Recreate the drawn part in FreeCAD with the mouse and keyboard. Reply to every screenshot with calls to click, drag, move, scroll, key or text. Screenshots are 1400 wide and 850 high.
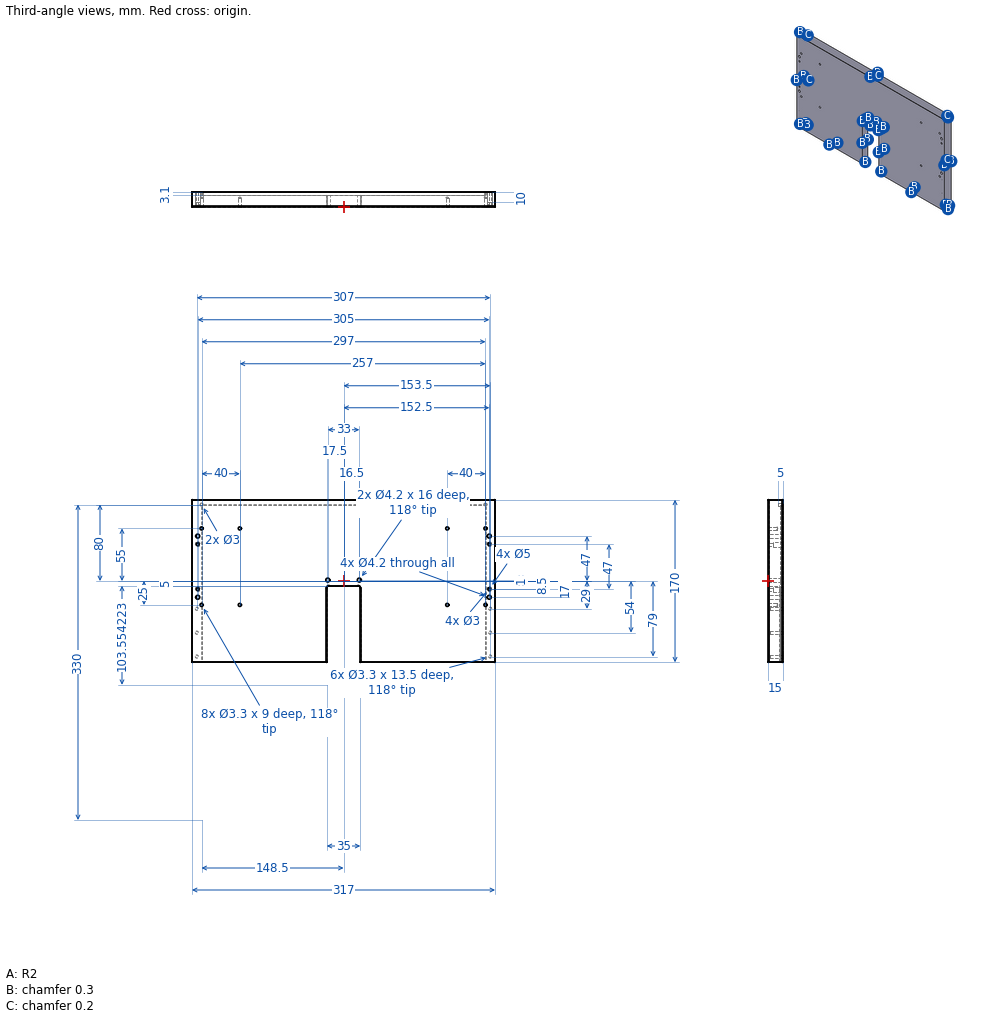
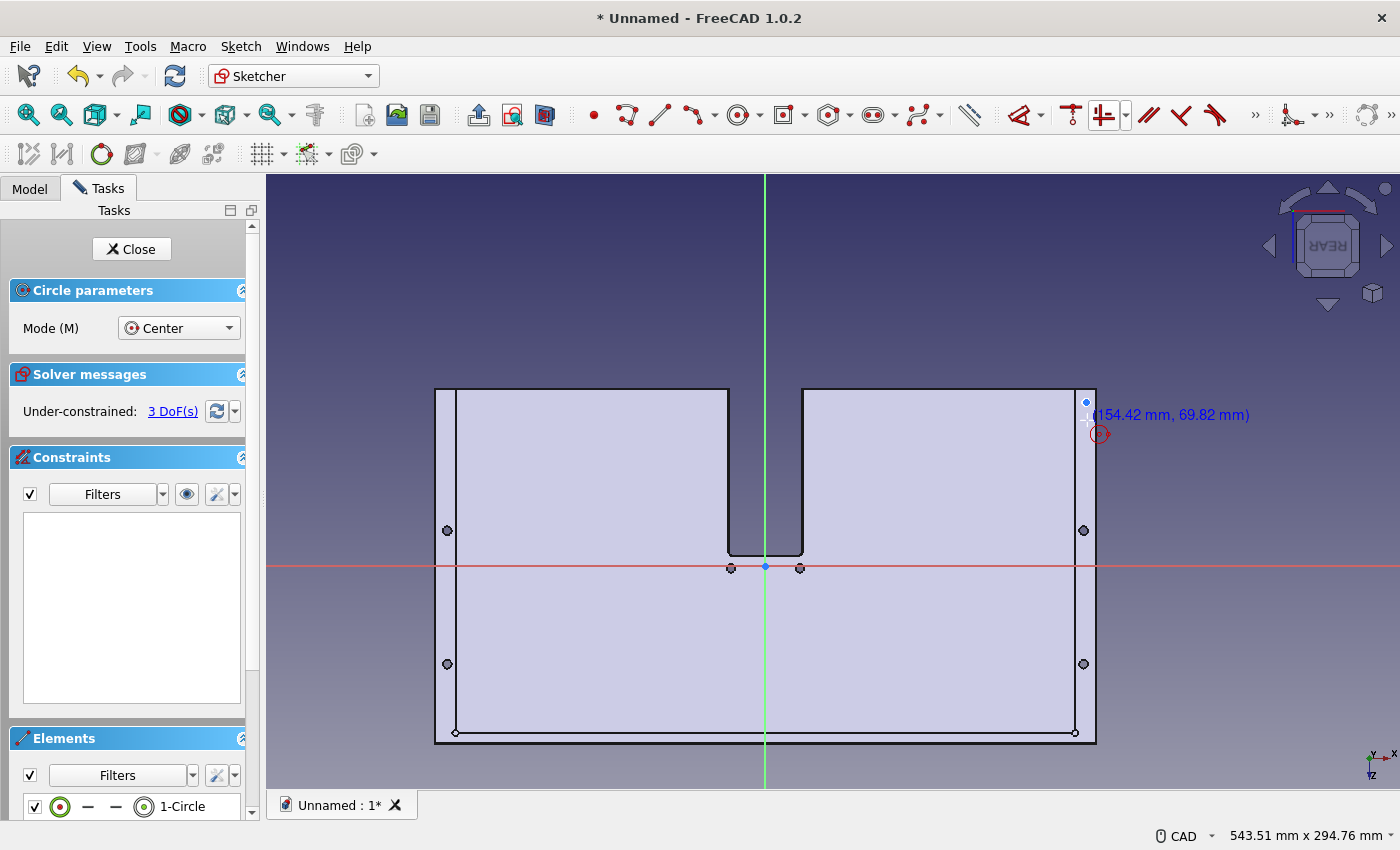
click(1086, 453)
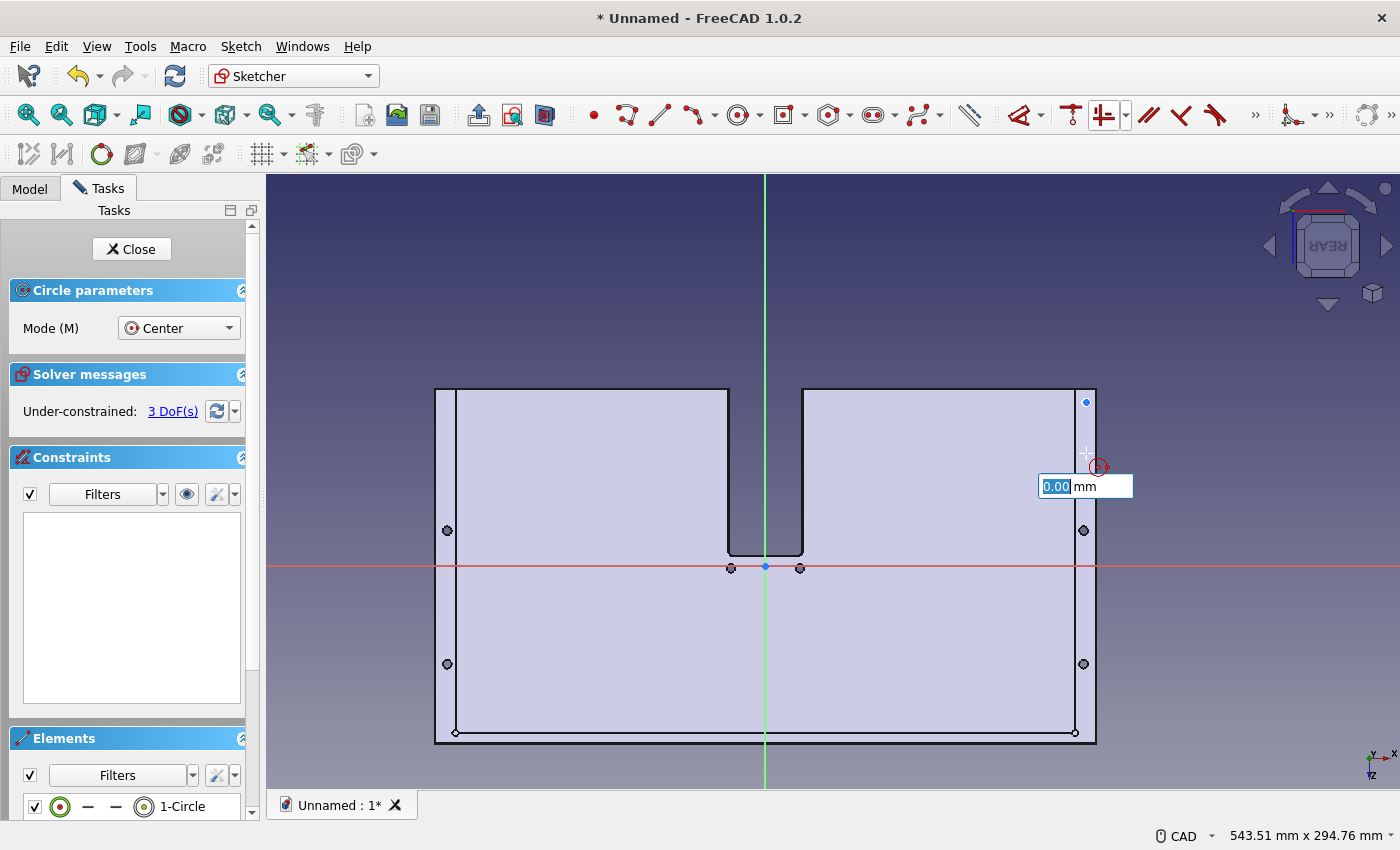
scroll(1088, 451, up, 8)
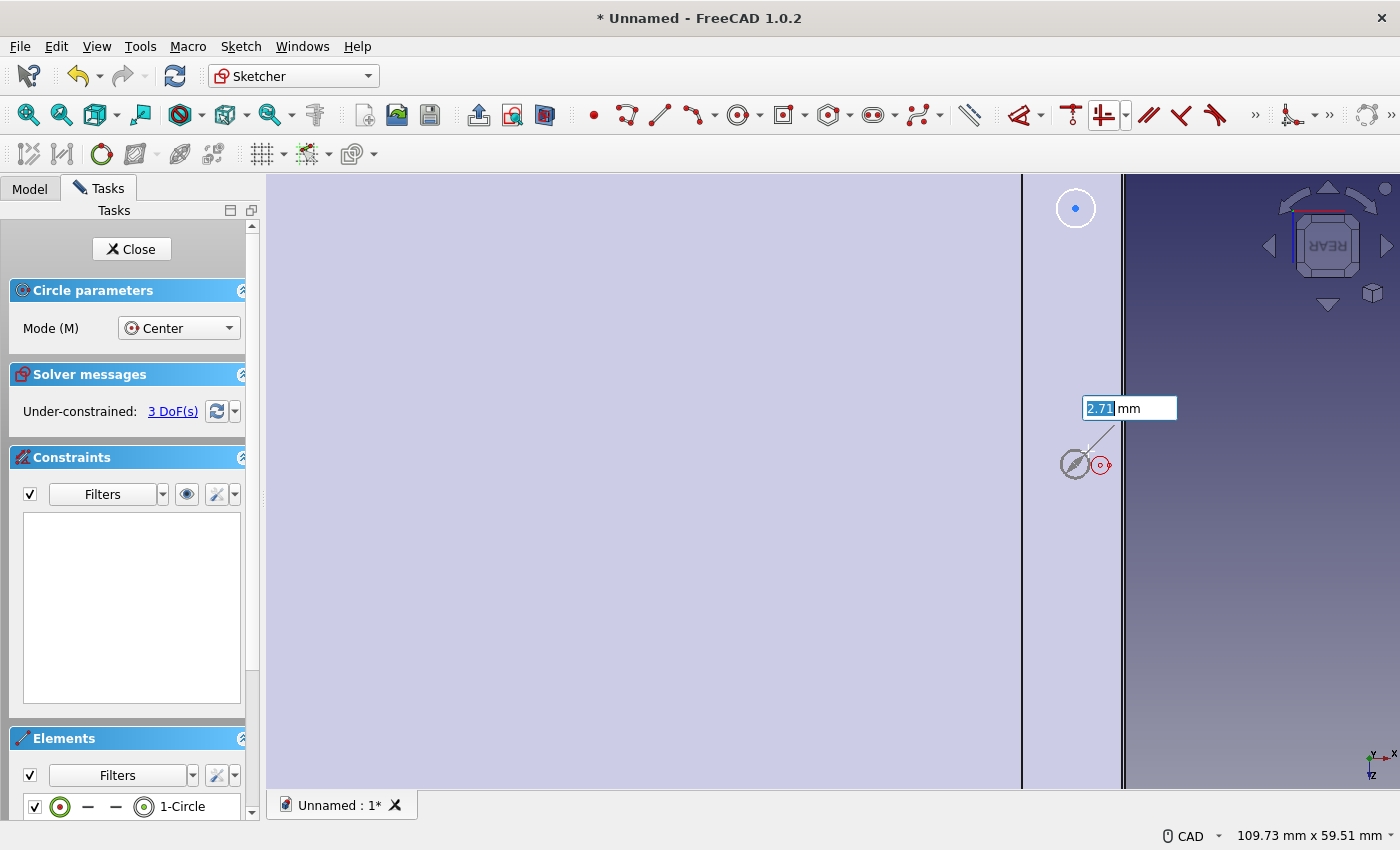
click(1086, 450)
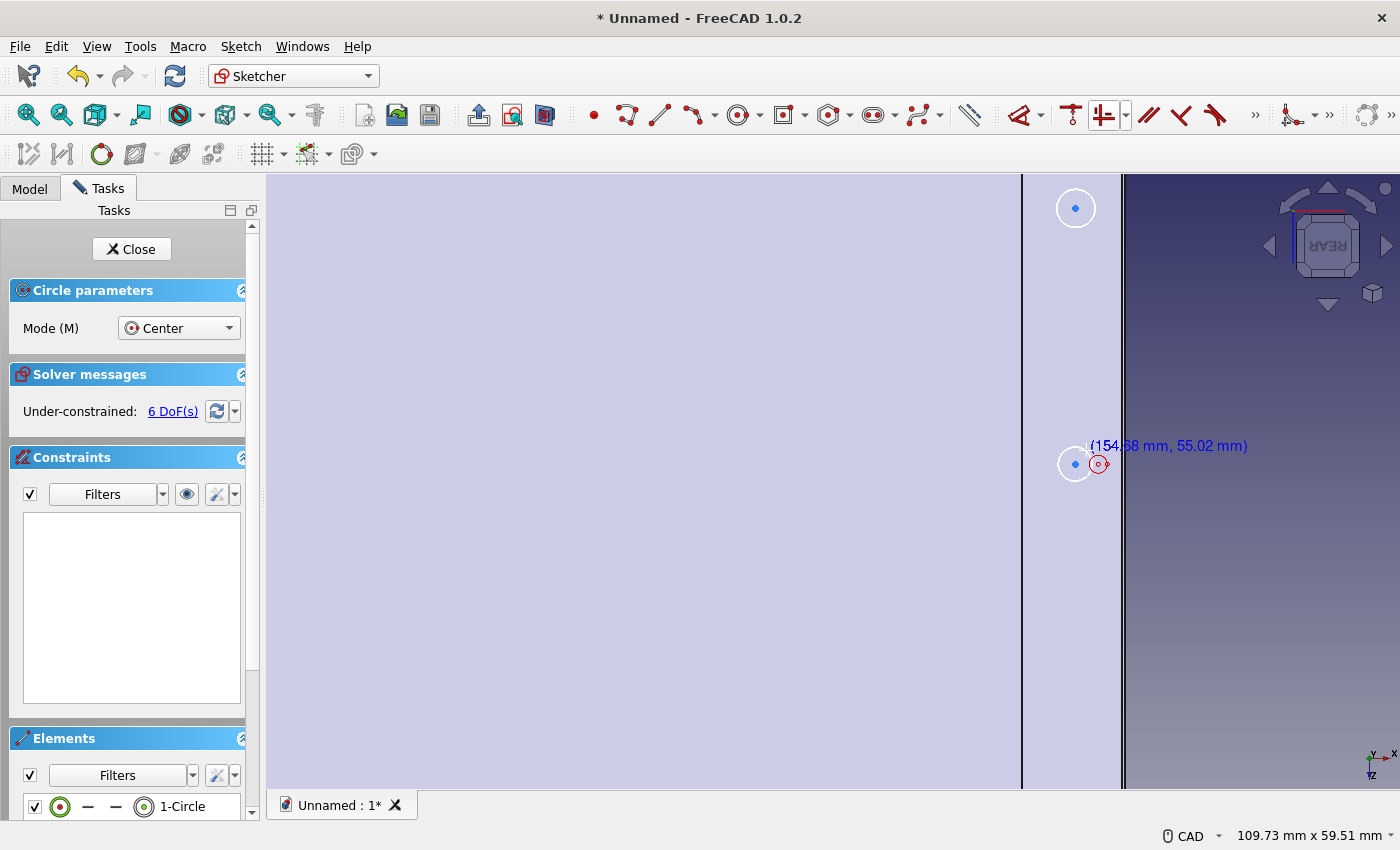
scroll(1074, 720, up, 2)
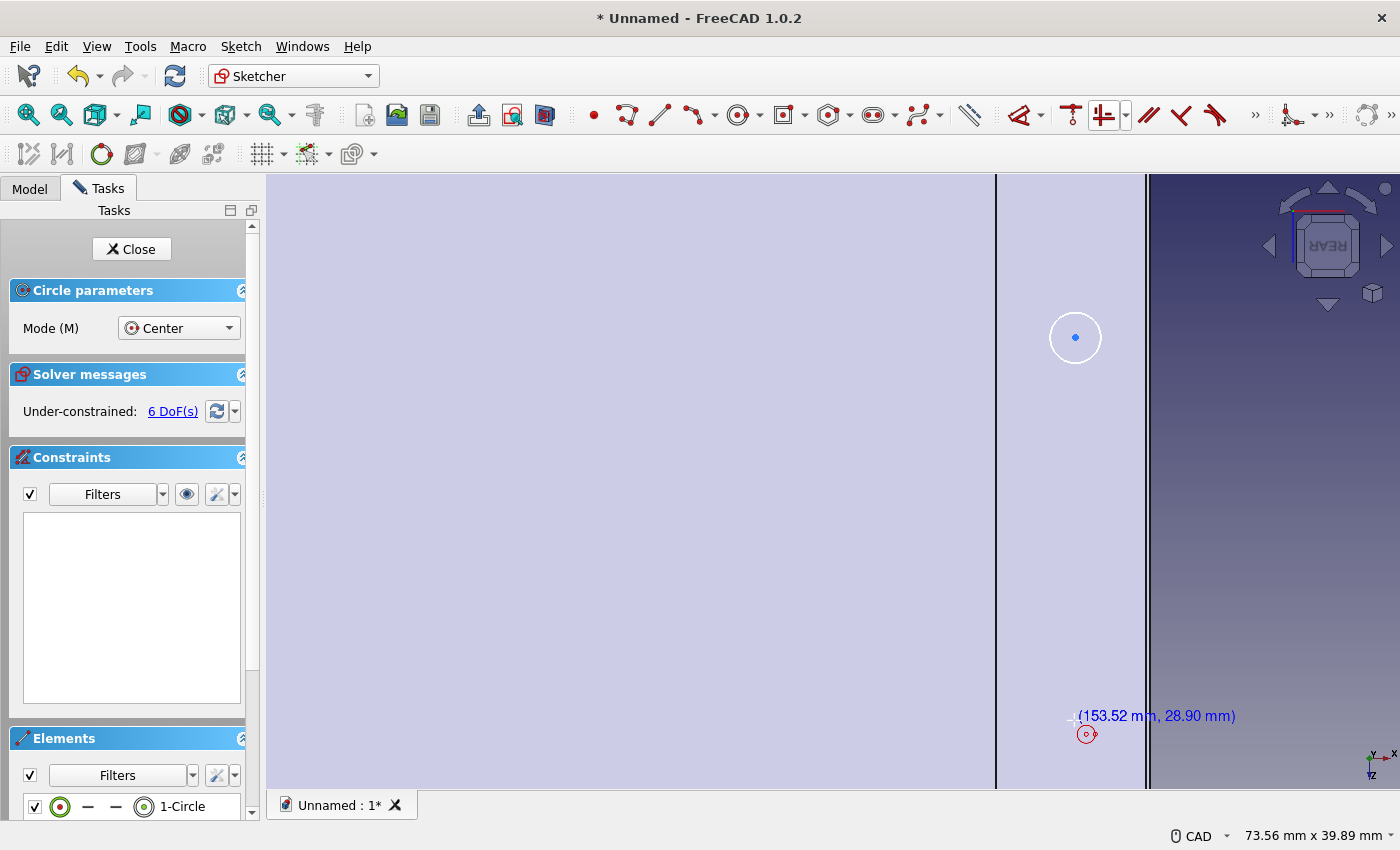
scroll(1087, 472, down, 10)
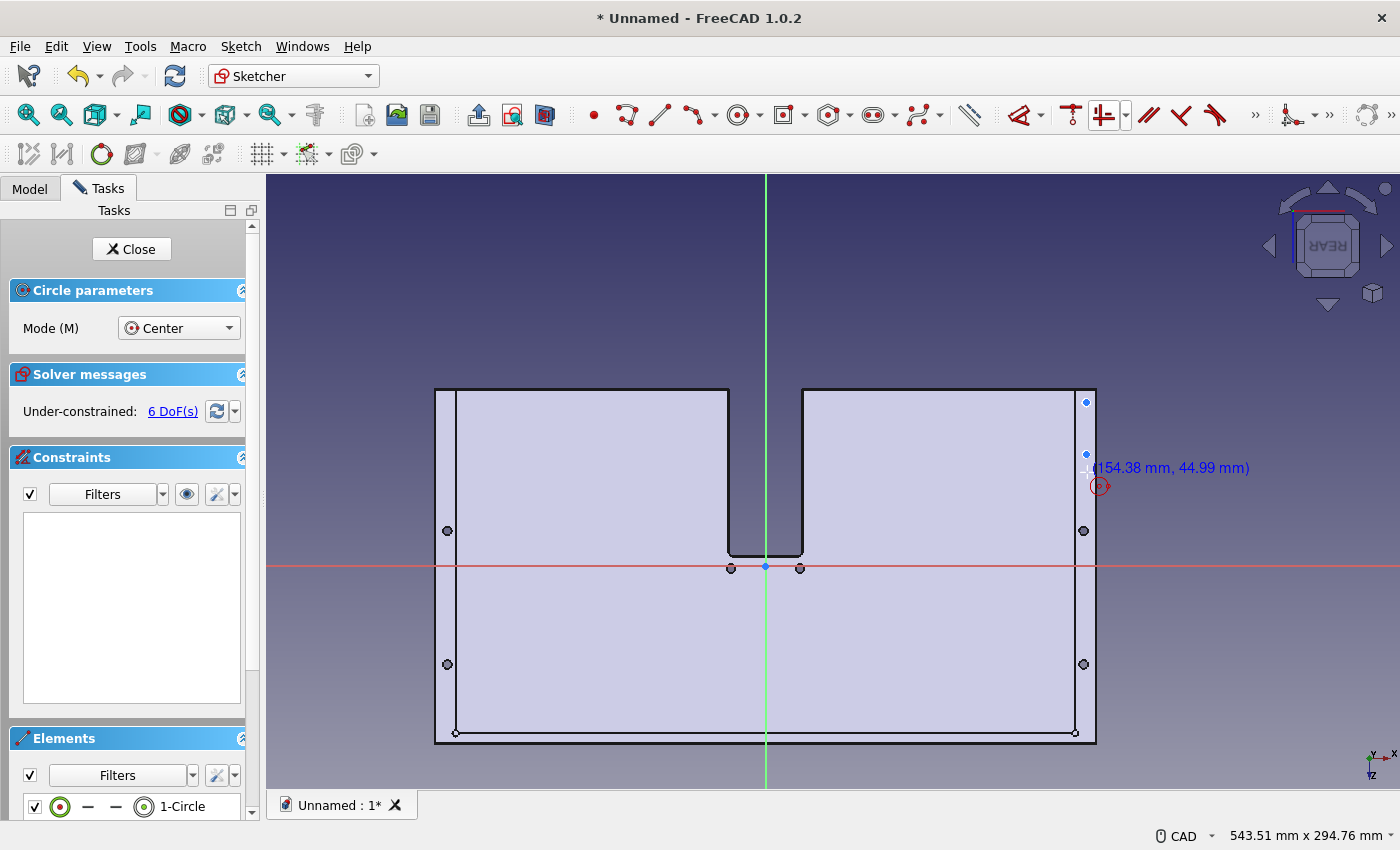
click(1086, 506)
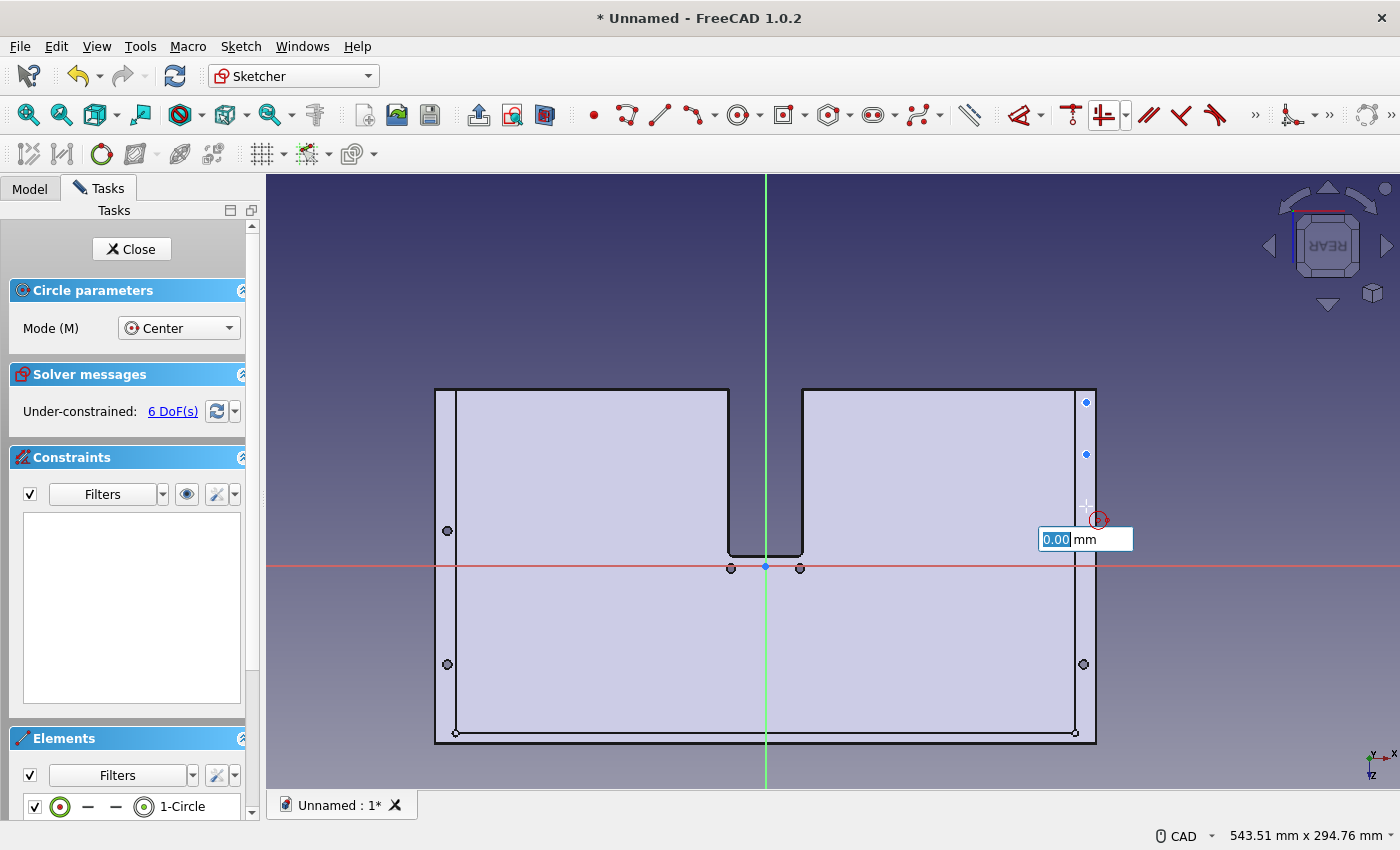
scroll(1088, 503, up, 8)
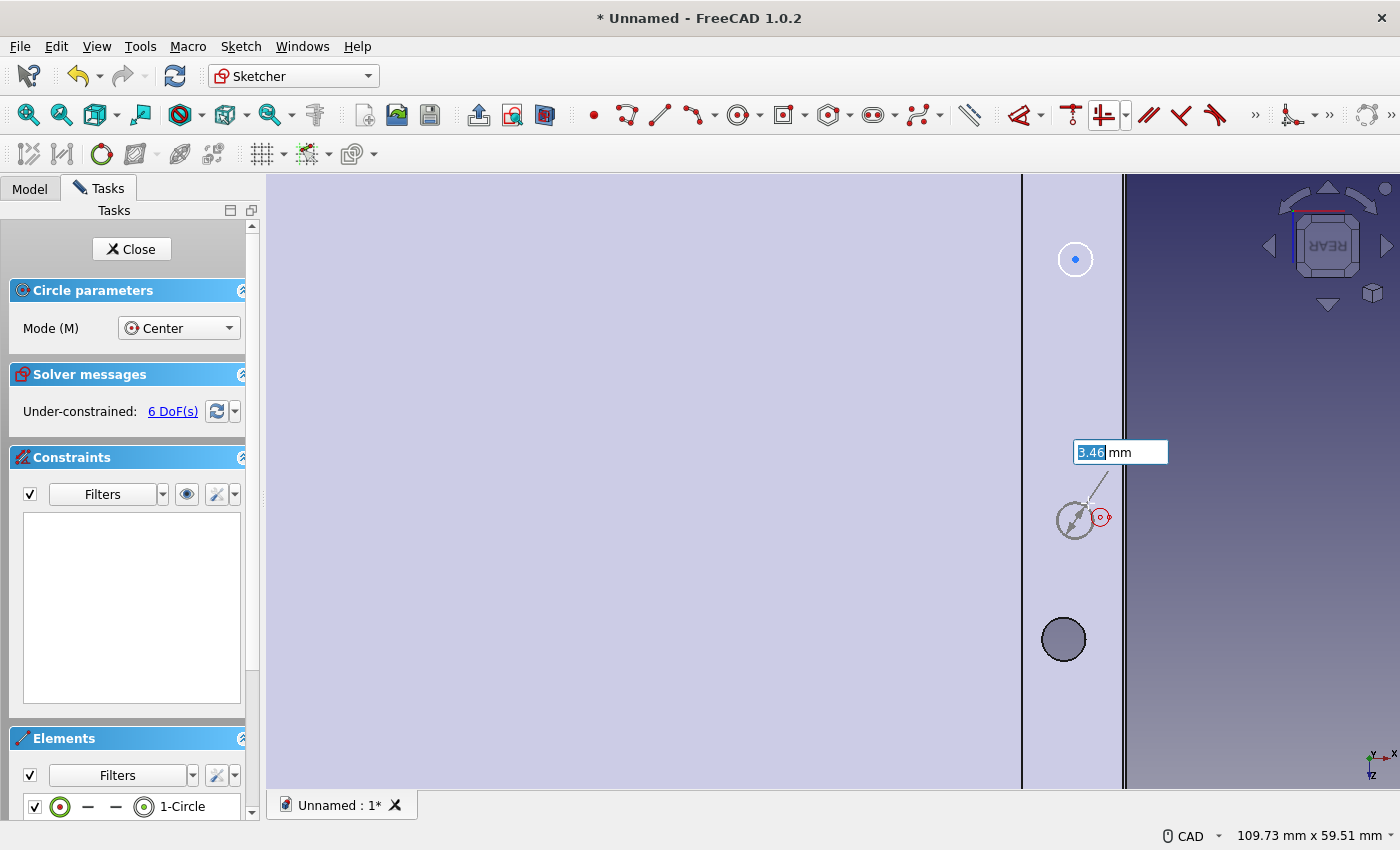
click(1086, 503)